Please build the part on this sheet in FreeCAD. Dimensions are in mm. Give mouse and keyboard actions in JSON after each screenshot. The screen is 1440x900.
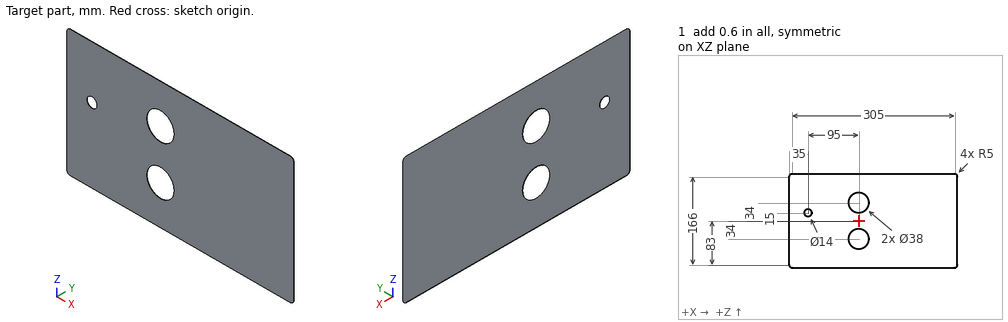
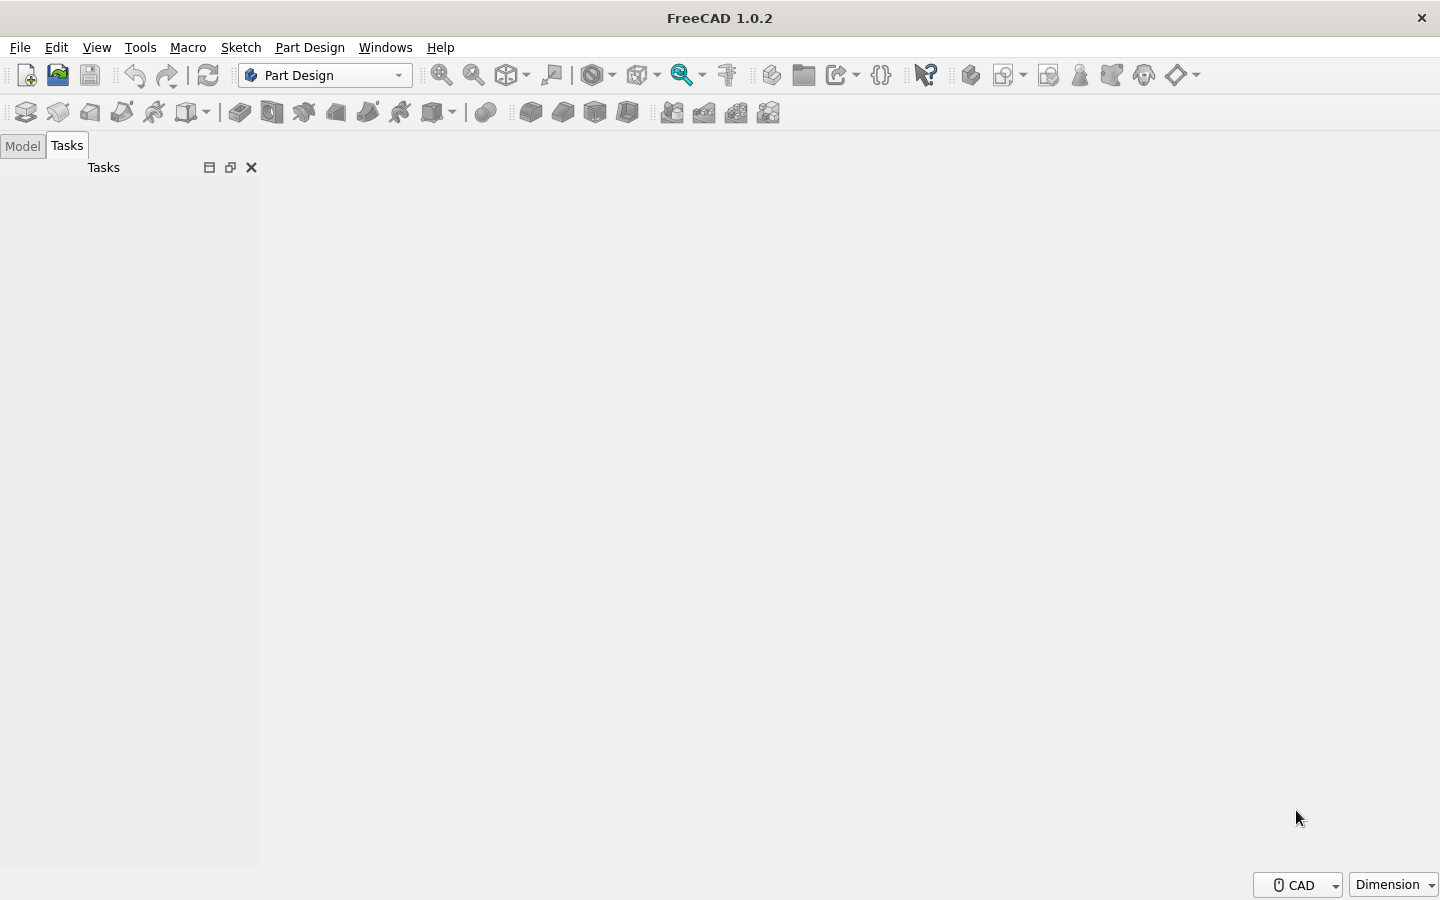
{"action": "left_click", "coordinate": [26, 76]}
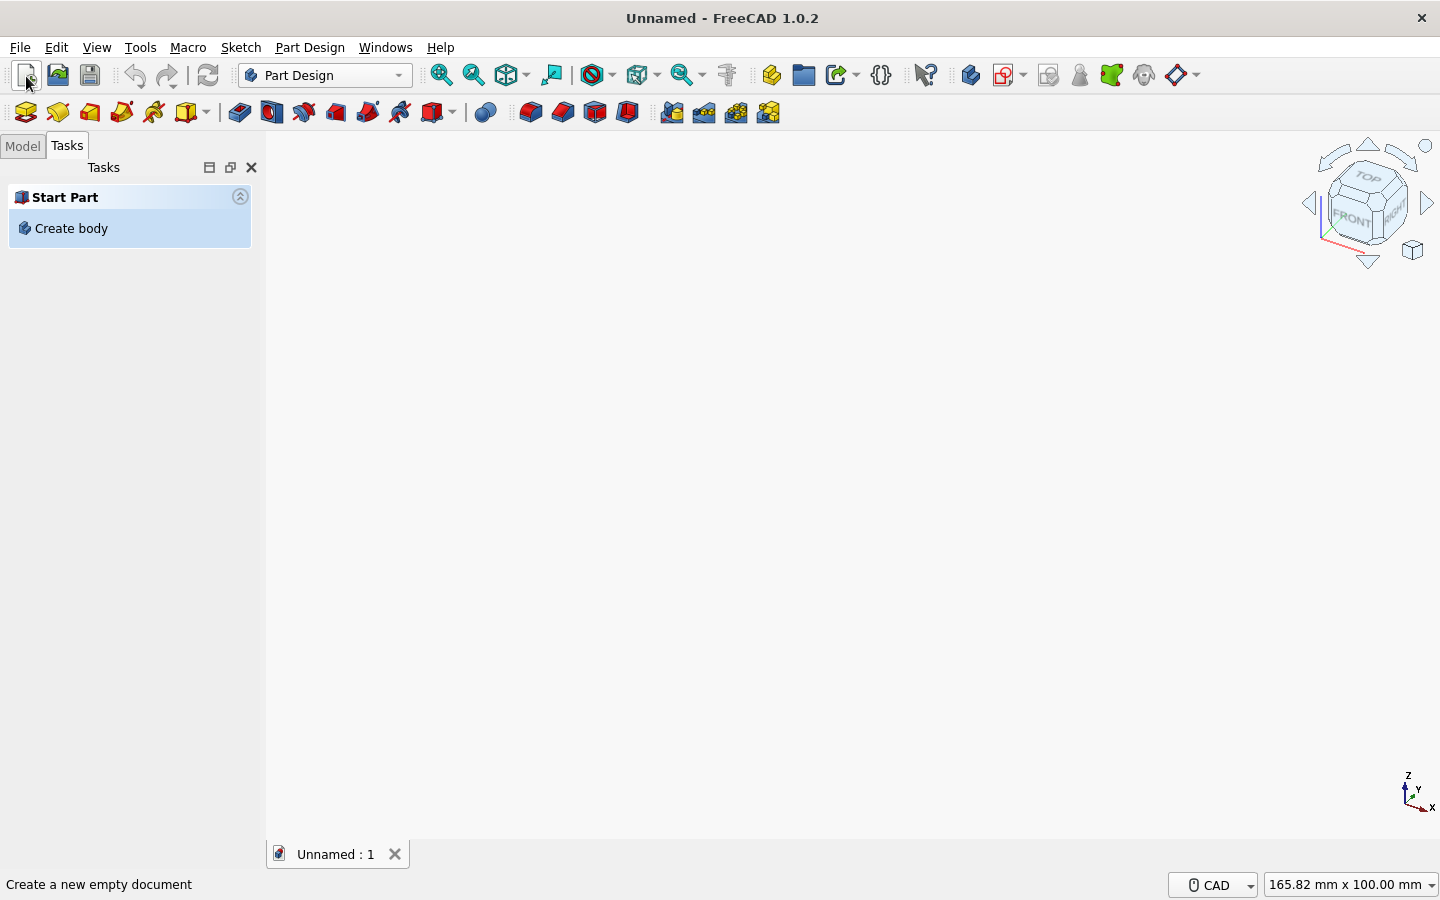
{"action": "left_click", "coordinate": [1004, 76]}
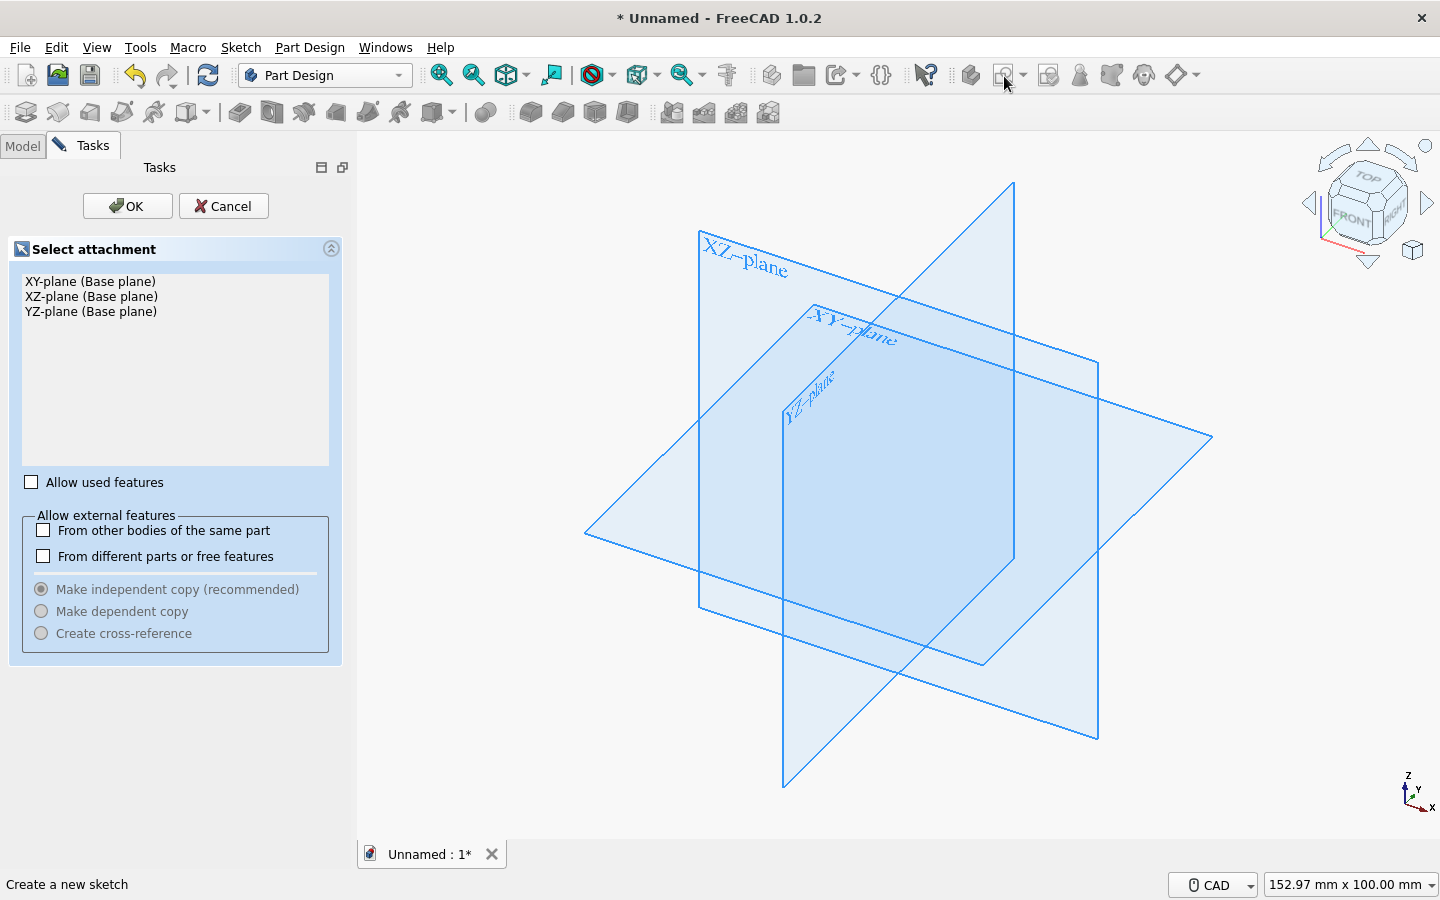
{"action": "left_click", "coordinate": [82, 296]}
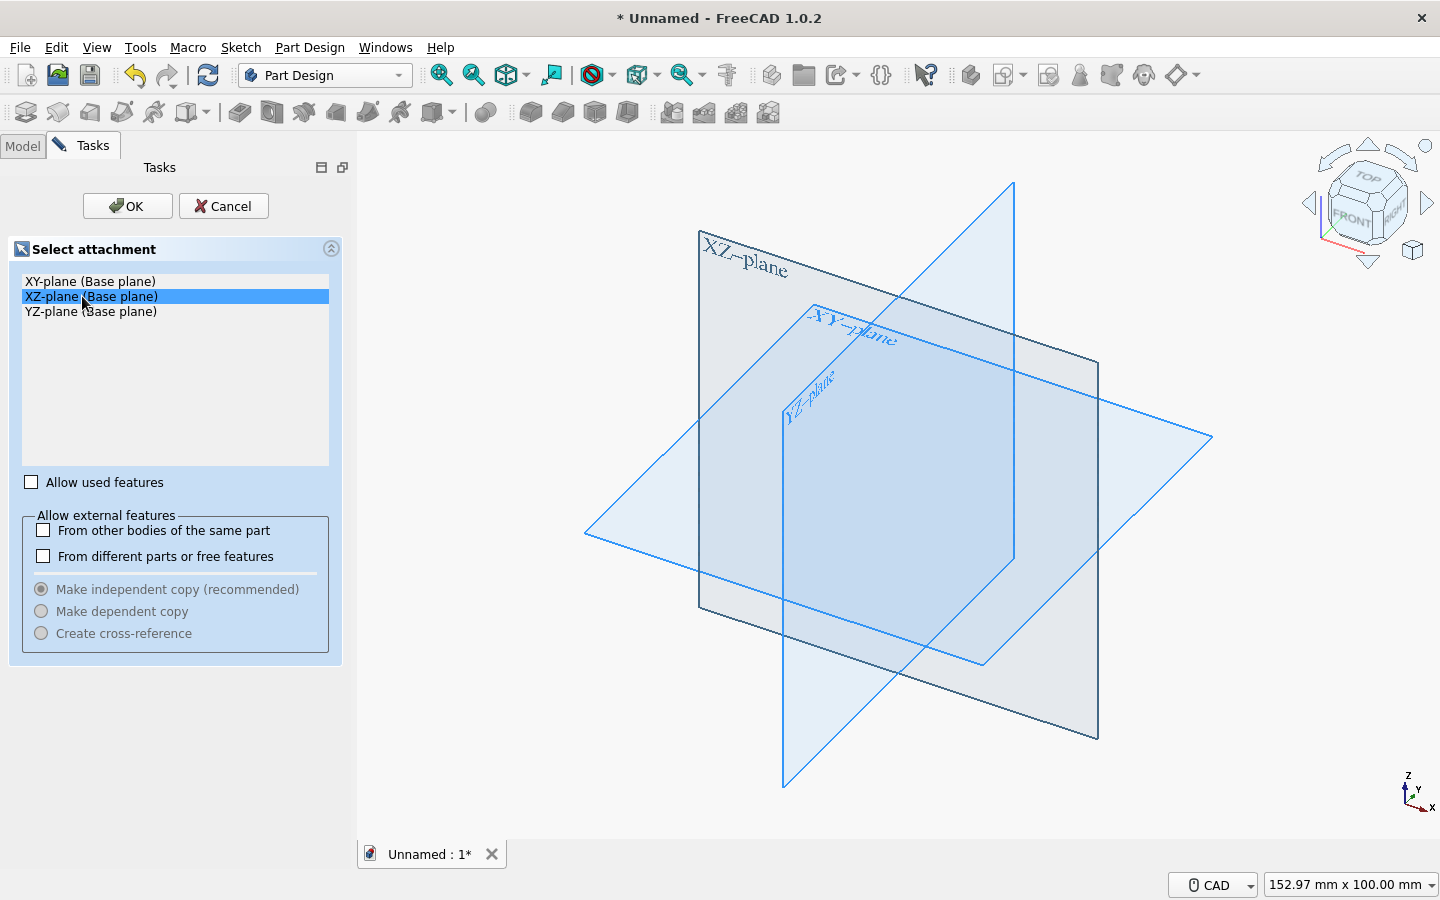
{"action": "left_click", "coordinate": [128, 206]}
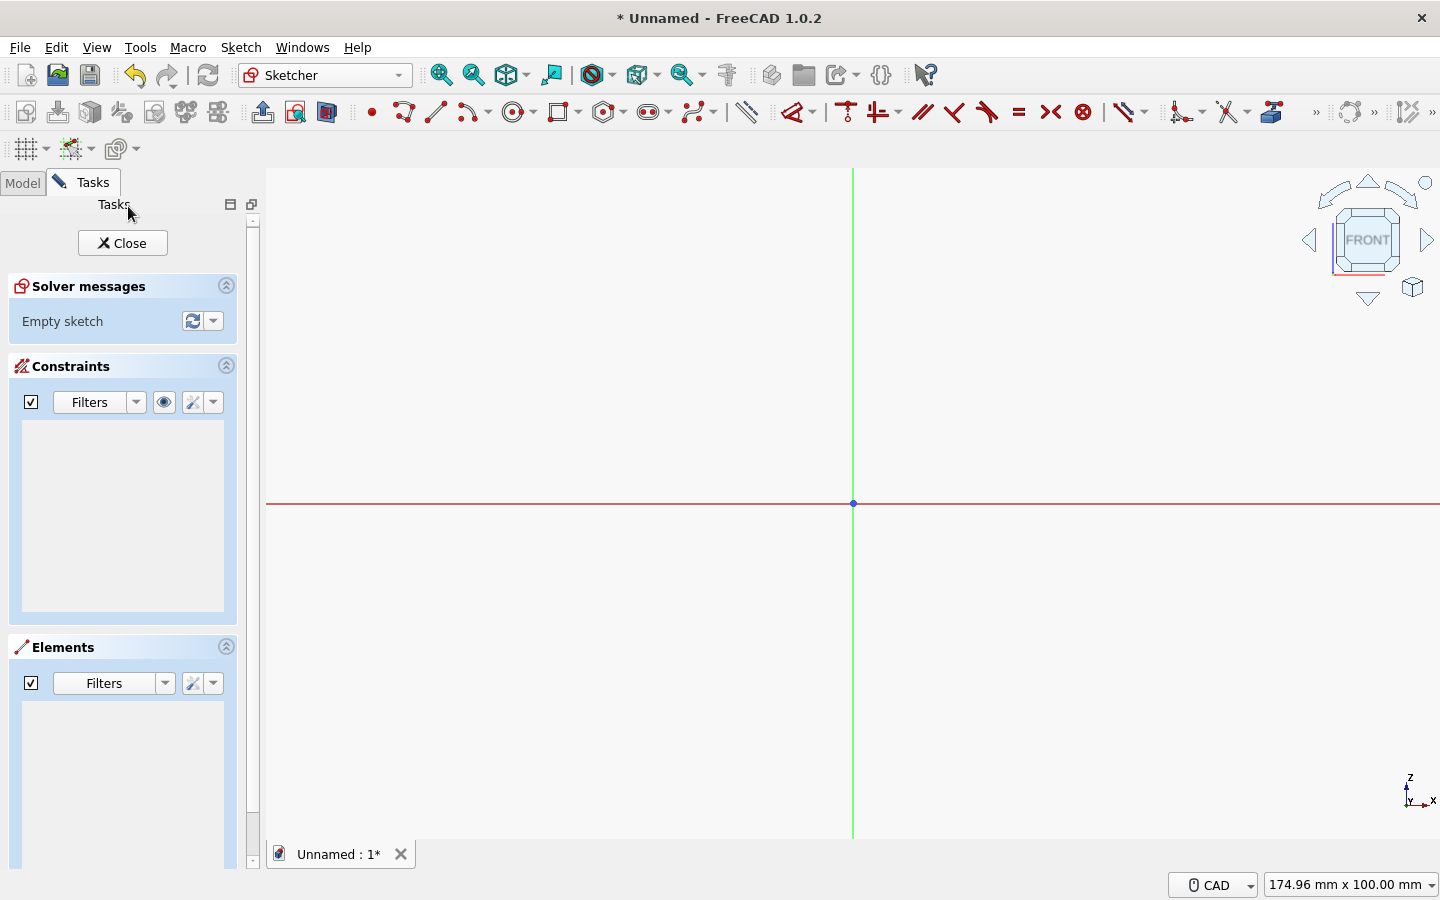
{"action": "scroll", "coordinate": [675, 504], "scroll_direction": "down", "scroll_amount": 6}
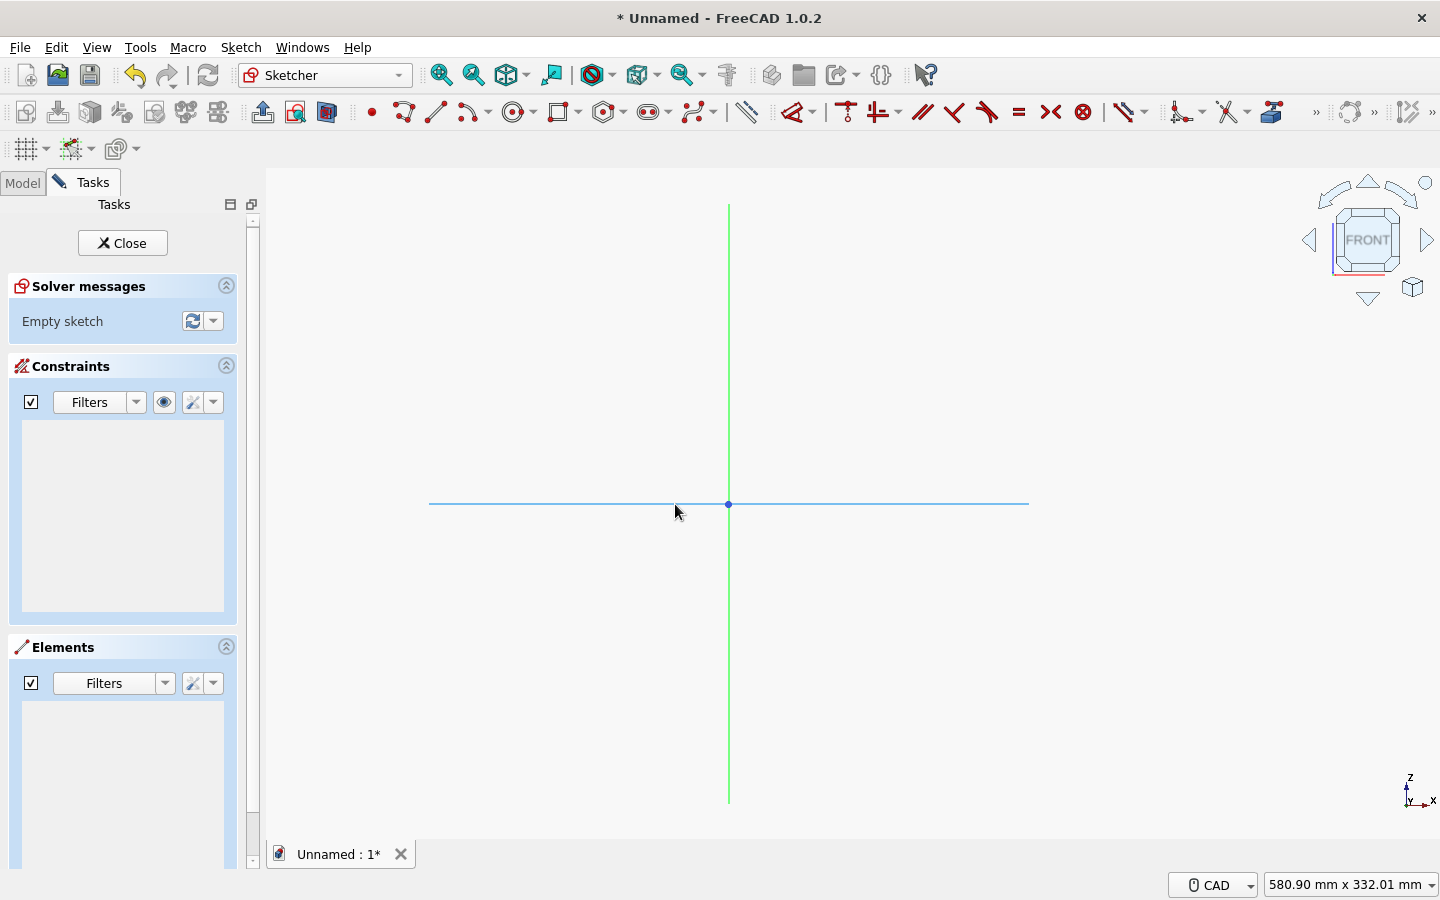
{"action": "left_click", "coordinate": [436, 112]}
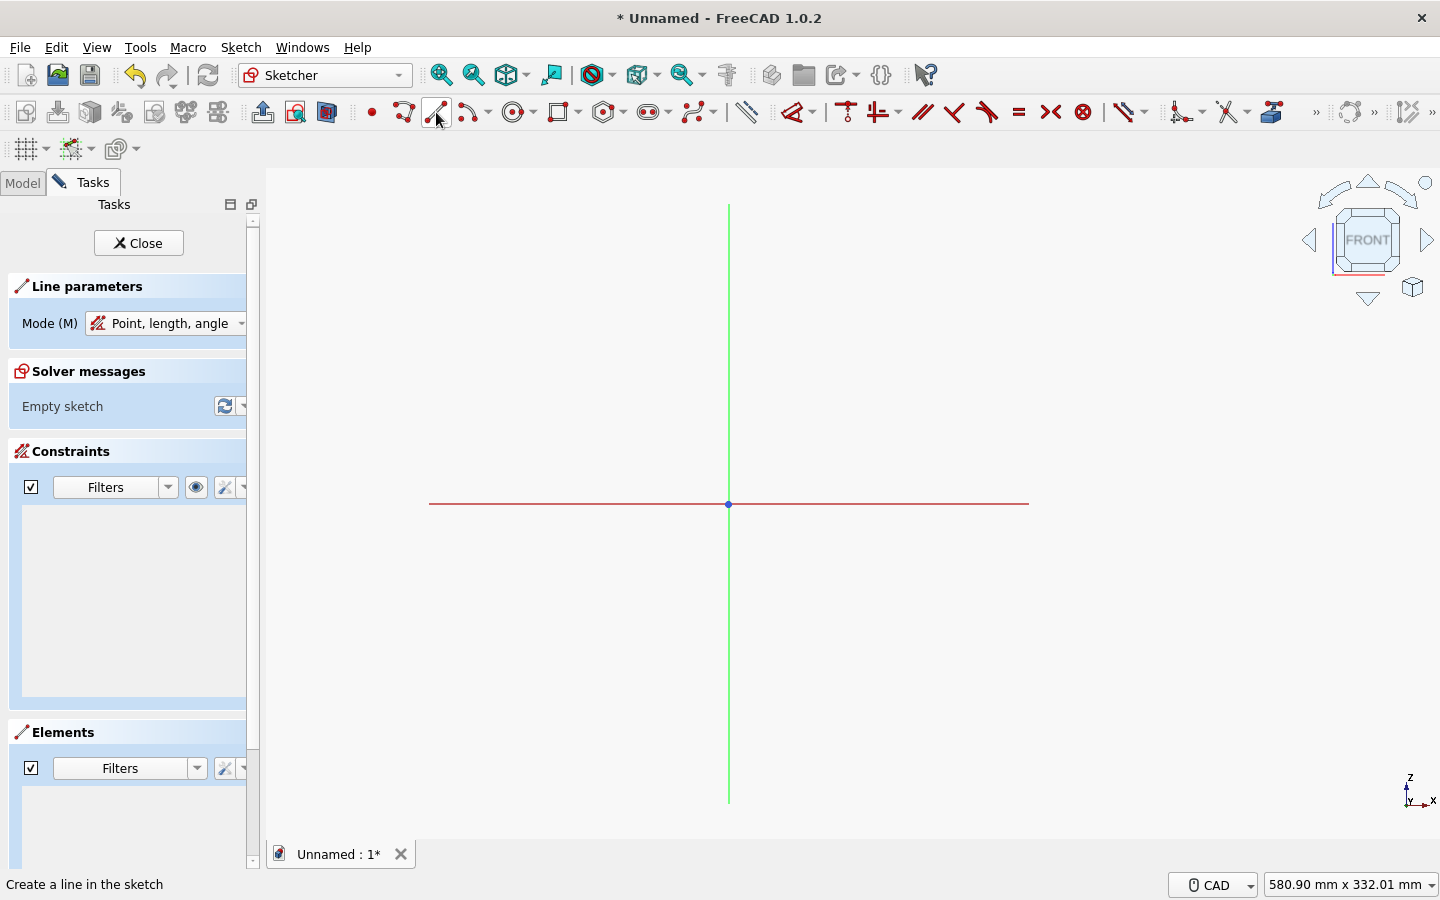
{"action": "left_click", "coordinate": [466, 672]}
{"action": "left_click", "coordinate": [466, 336]}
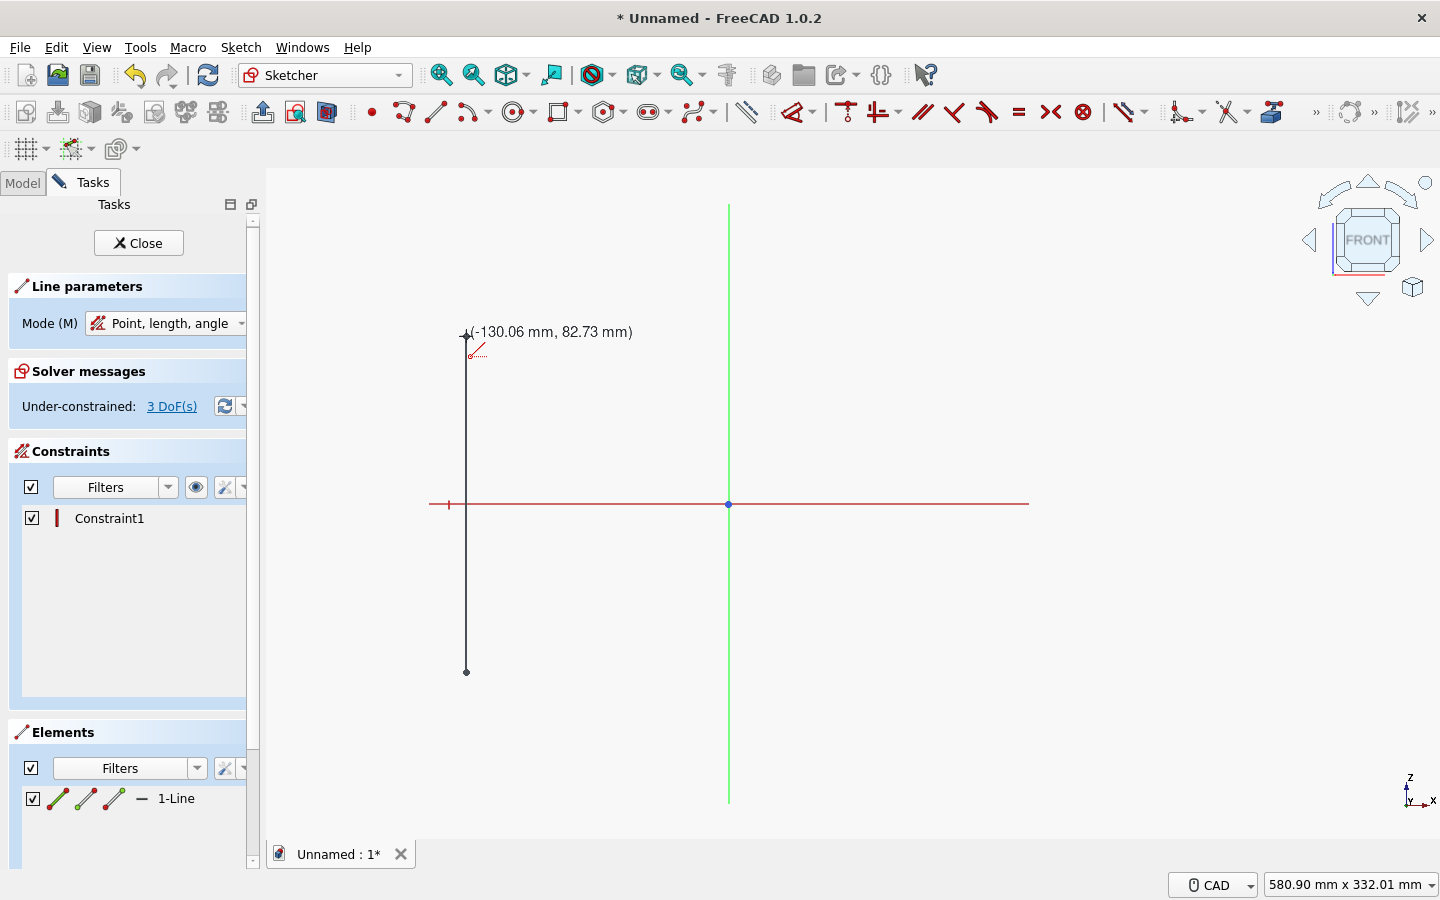
{"action": "left_click", "coordinate": [476, 326]}
{"action": "left_click", "coordinate": [1093, 326]}